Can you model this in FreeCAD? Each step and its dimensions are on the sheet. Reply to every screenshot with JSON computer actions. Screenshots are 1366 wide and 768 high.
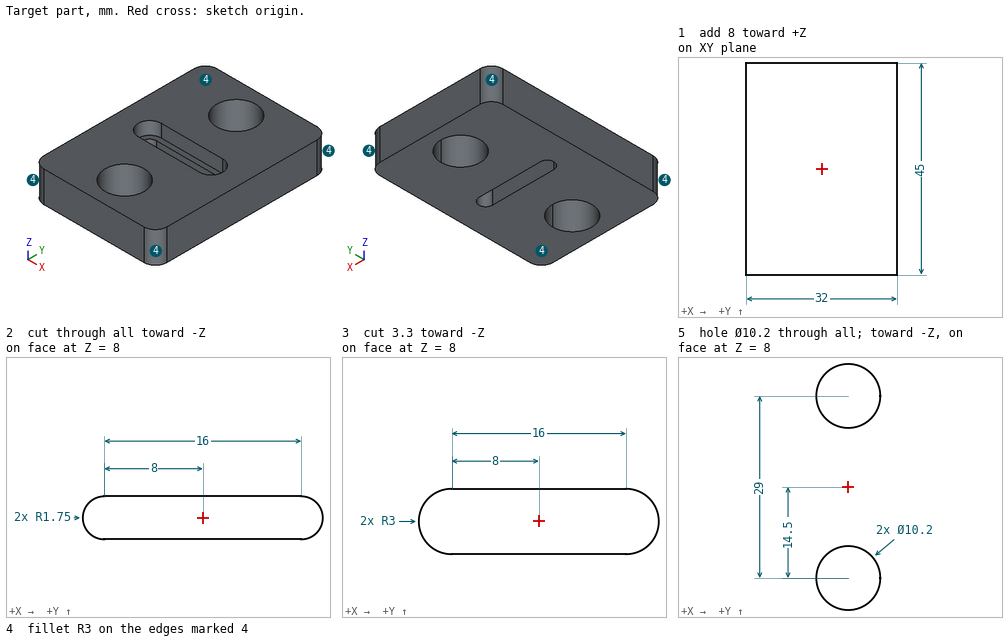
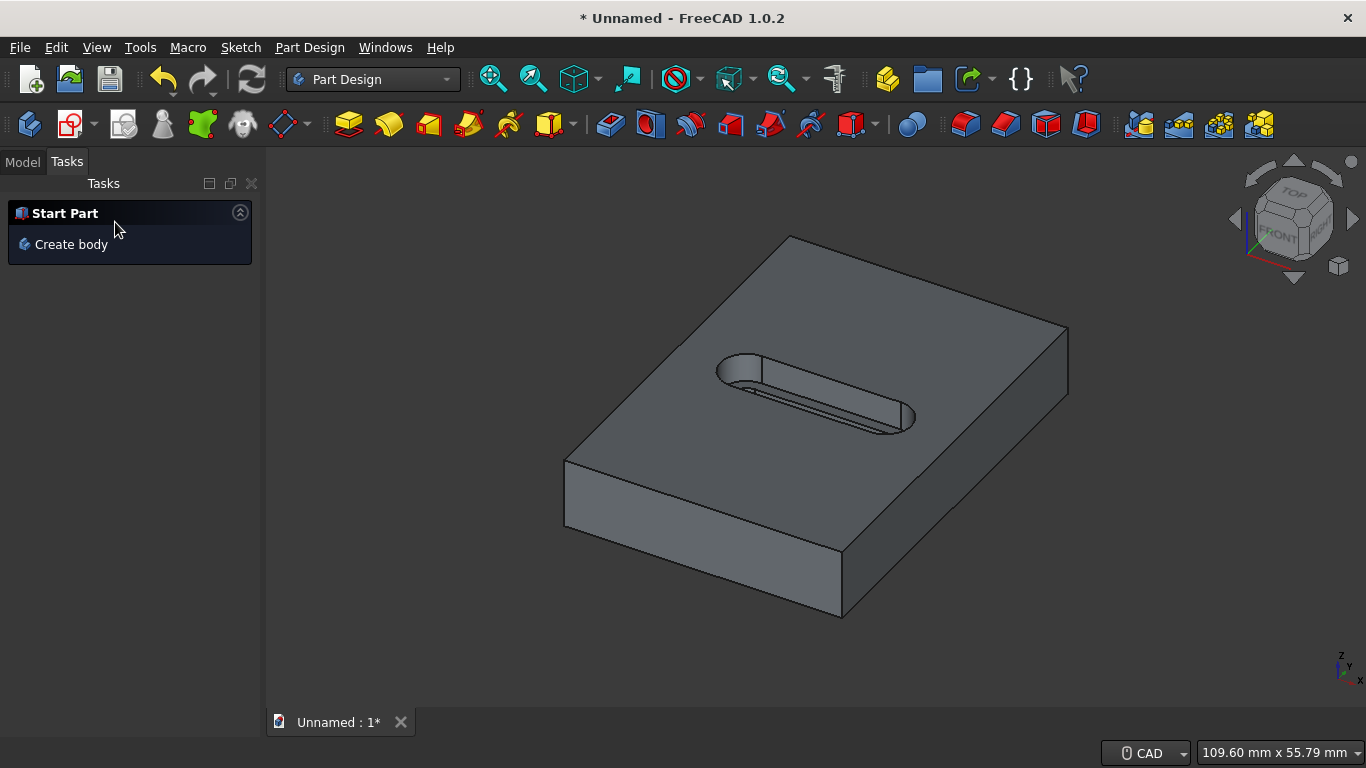
{"action": "left_click", "coordinate": [842, 584]}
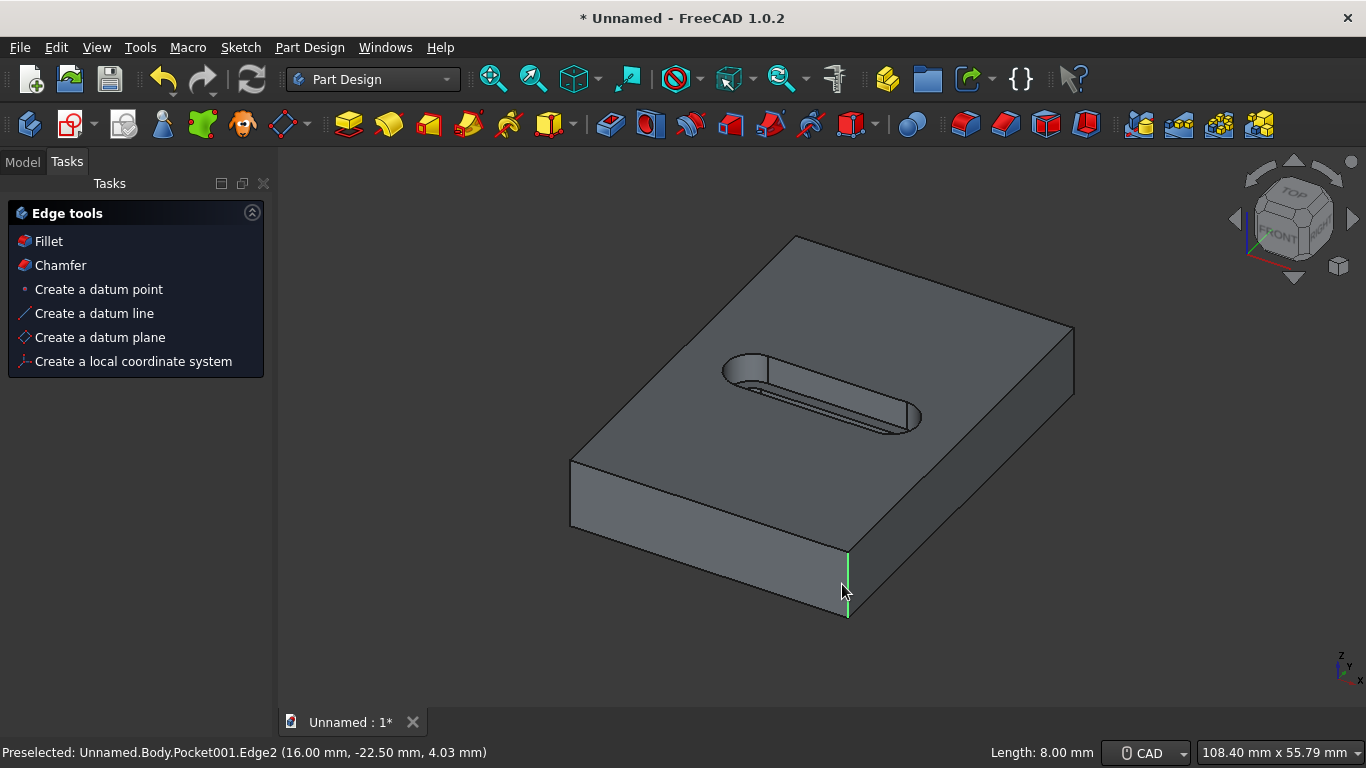
{"action": "key", "text": "0"}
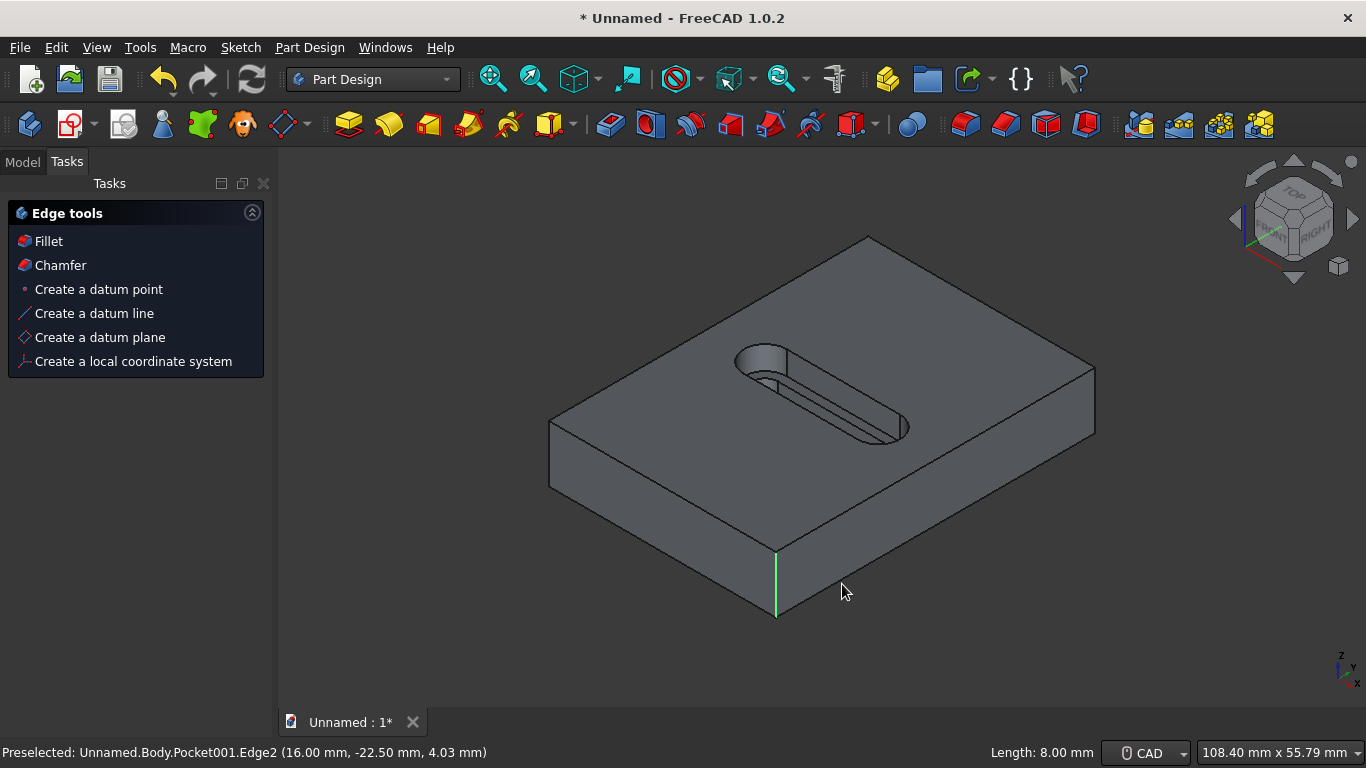
{"action": "key", "text": "2"}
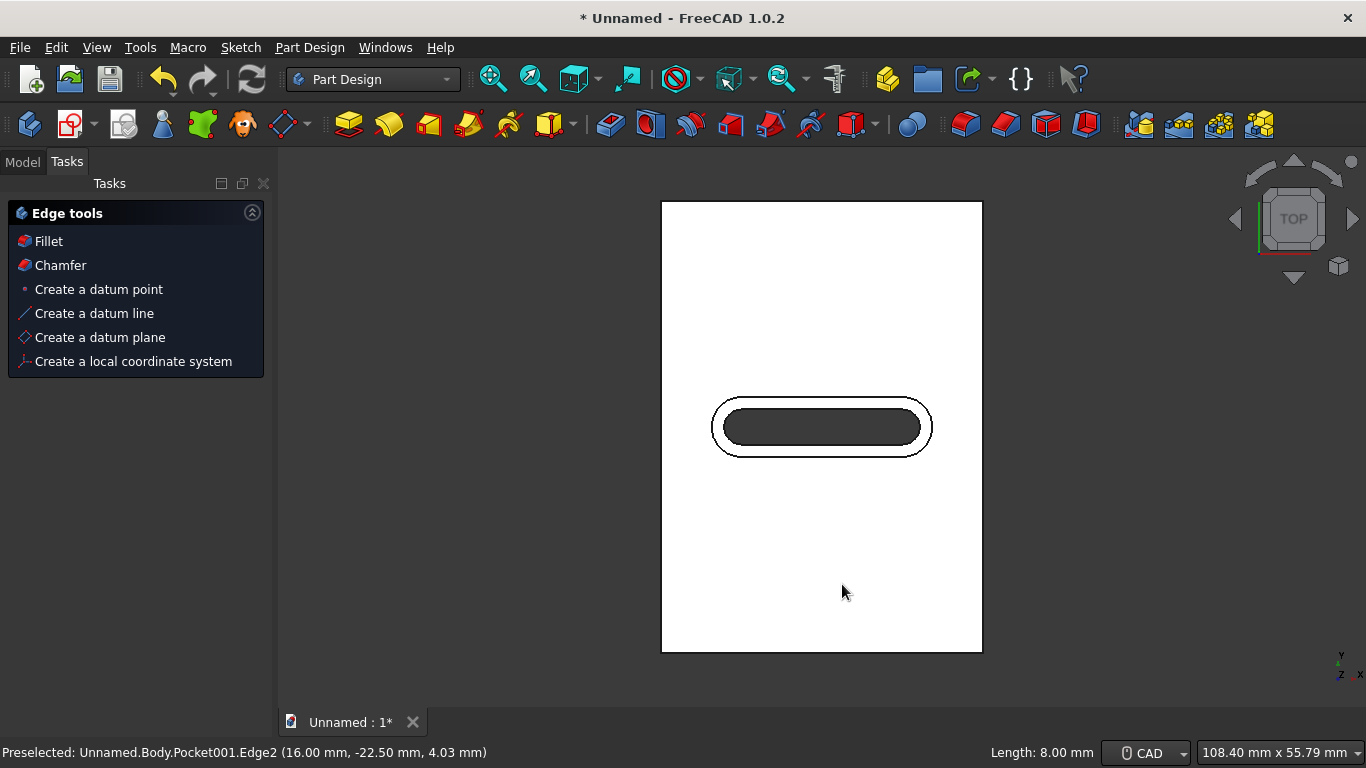
{"action": "key", "text": "1"}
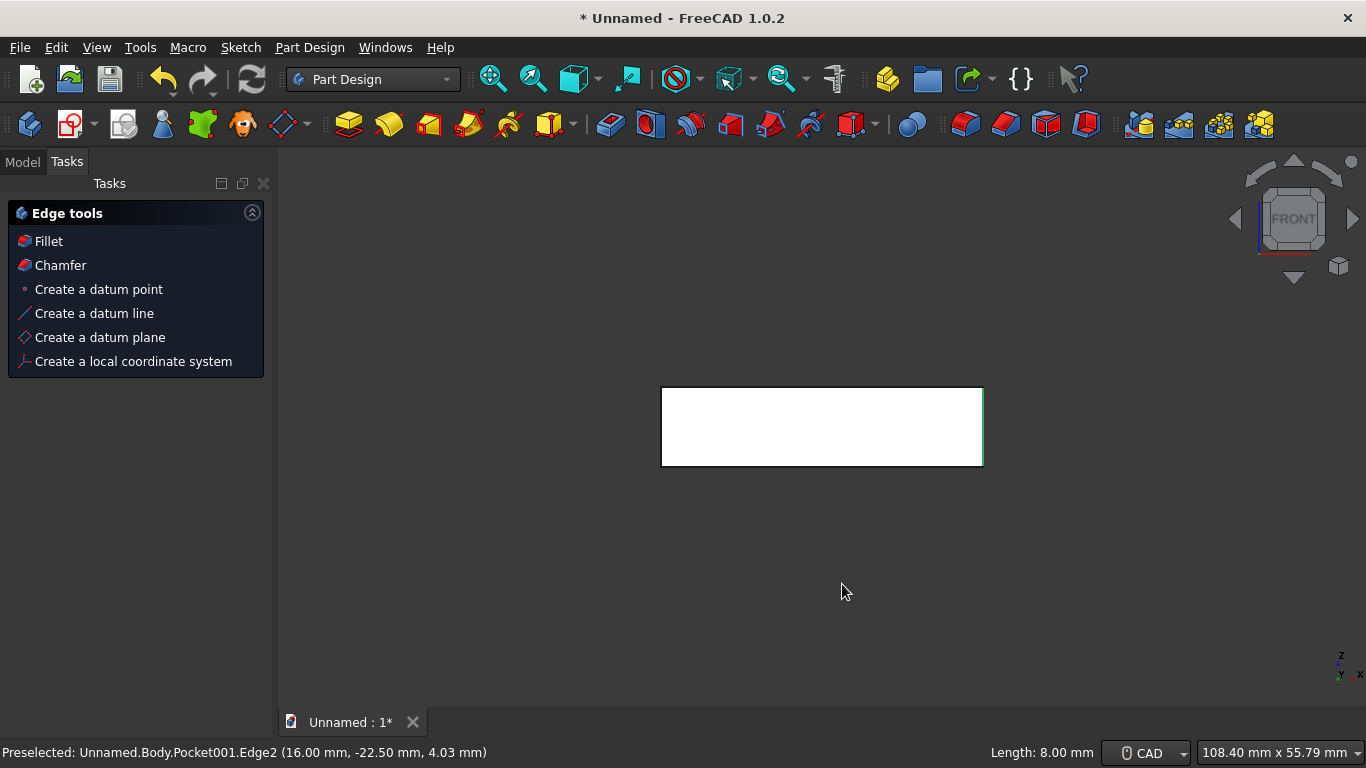
{"action": "key", "text": "v f"}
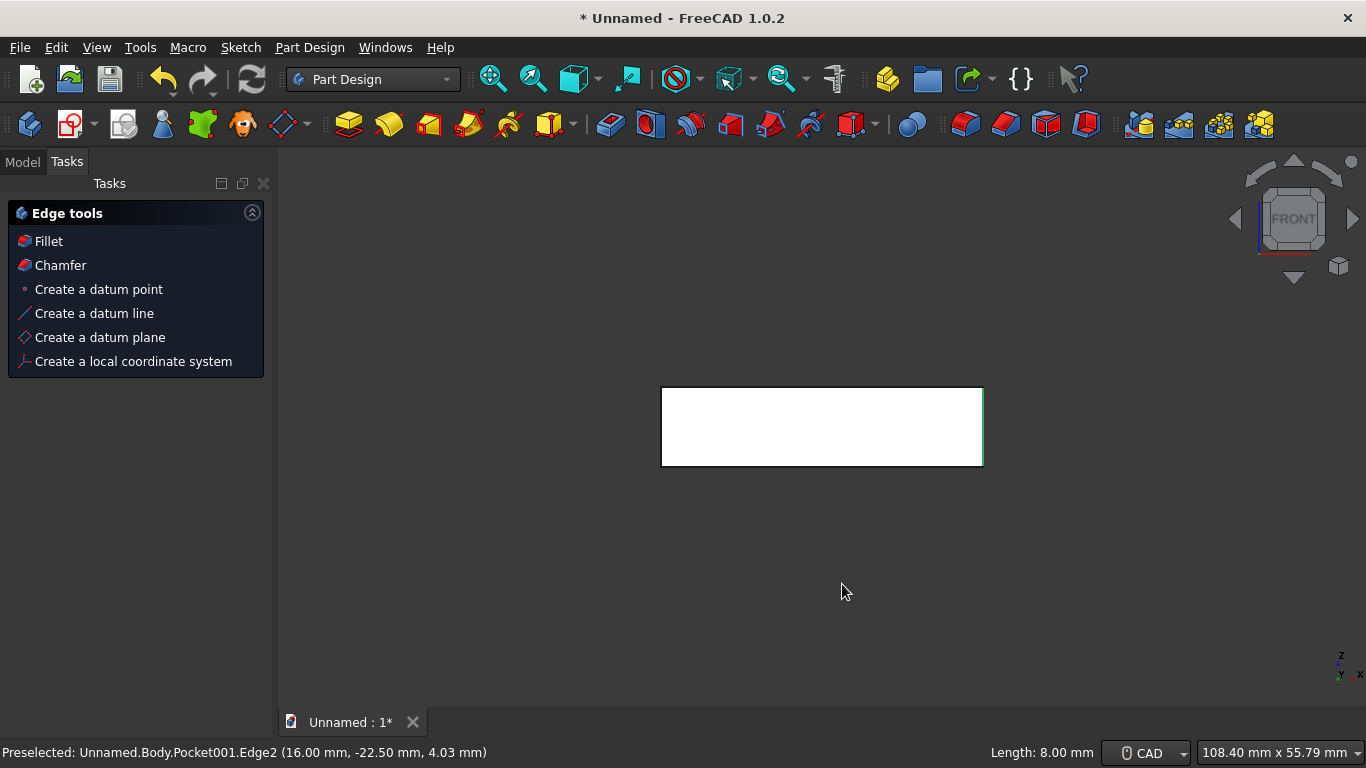
{"action": "left_click", "coordinate": [661, 426], "text": "ctrl"}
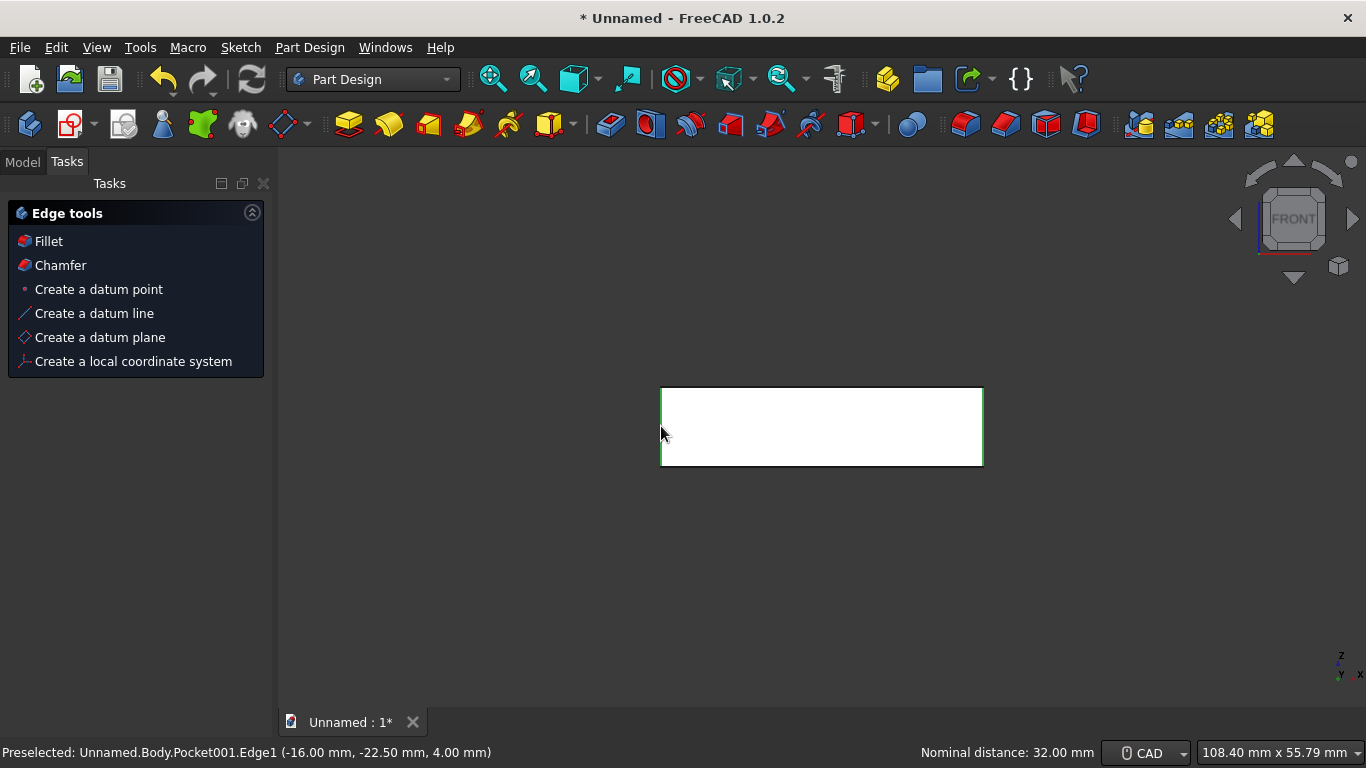
{"action": "key", "text": "3"}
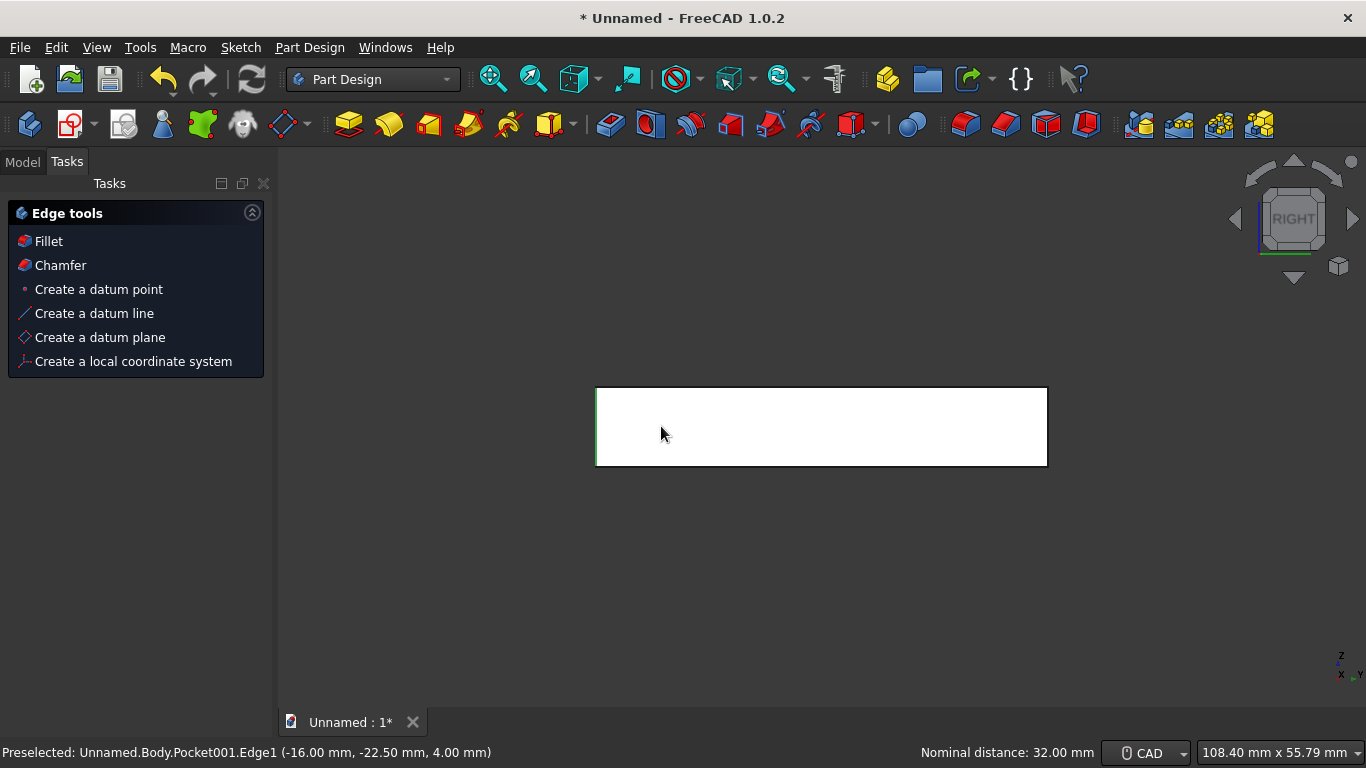
{"action": "key", "text": "v f"}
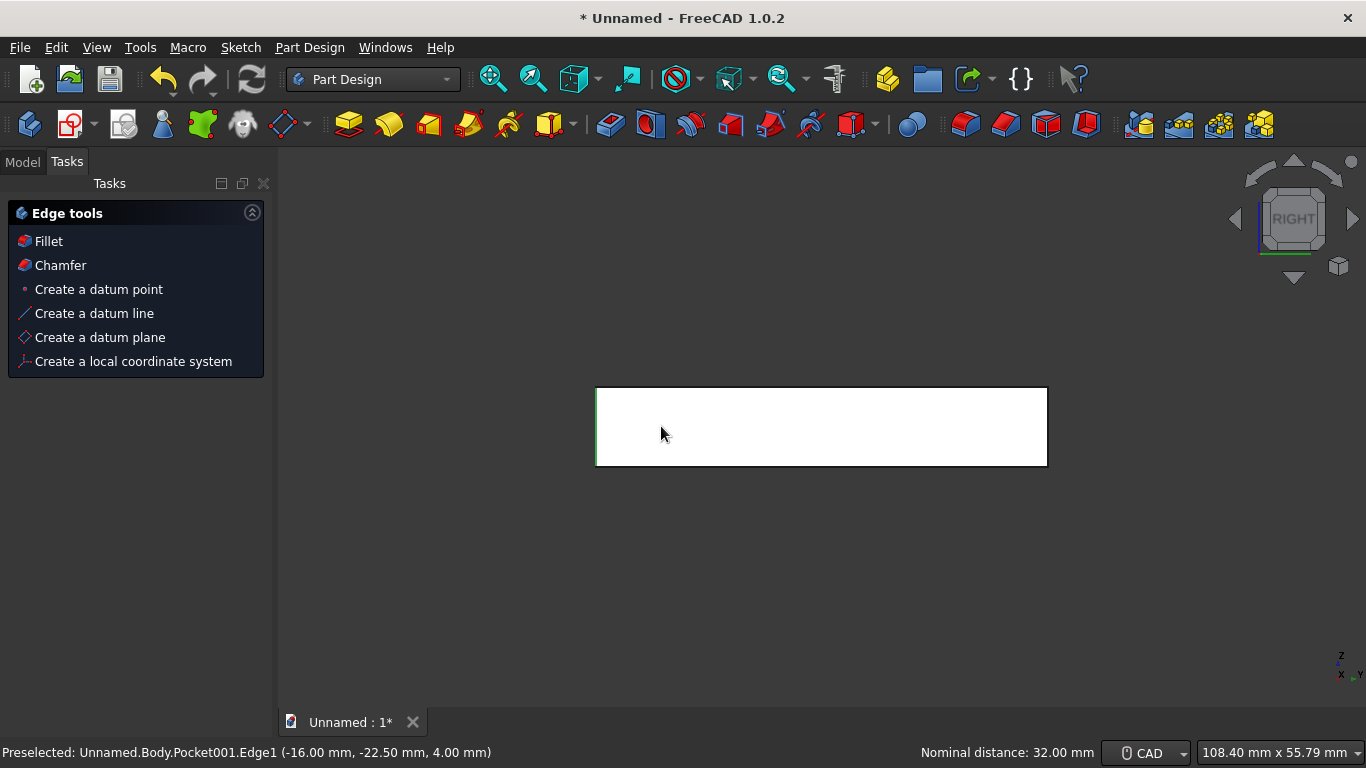
{"action": "left_click", "coordinate": [1048, 426], "text": "ctrl"}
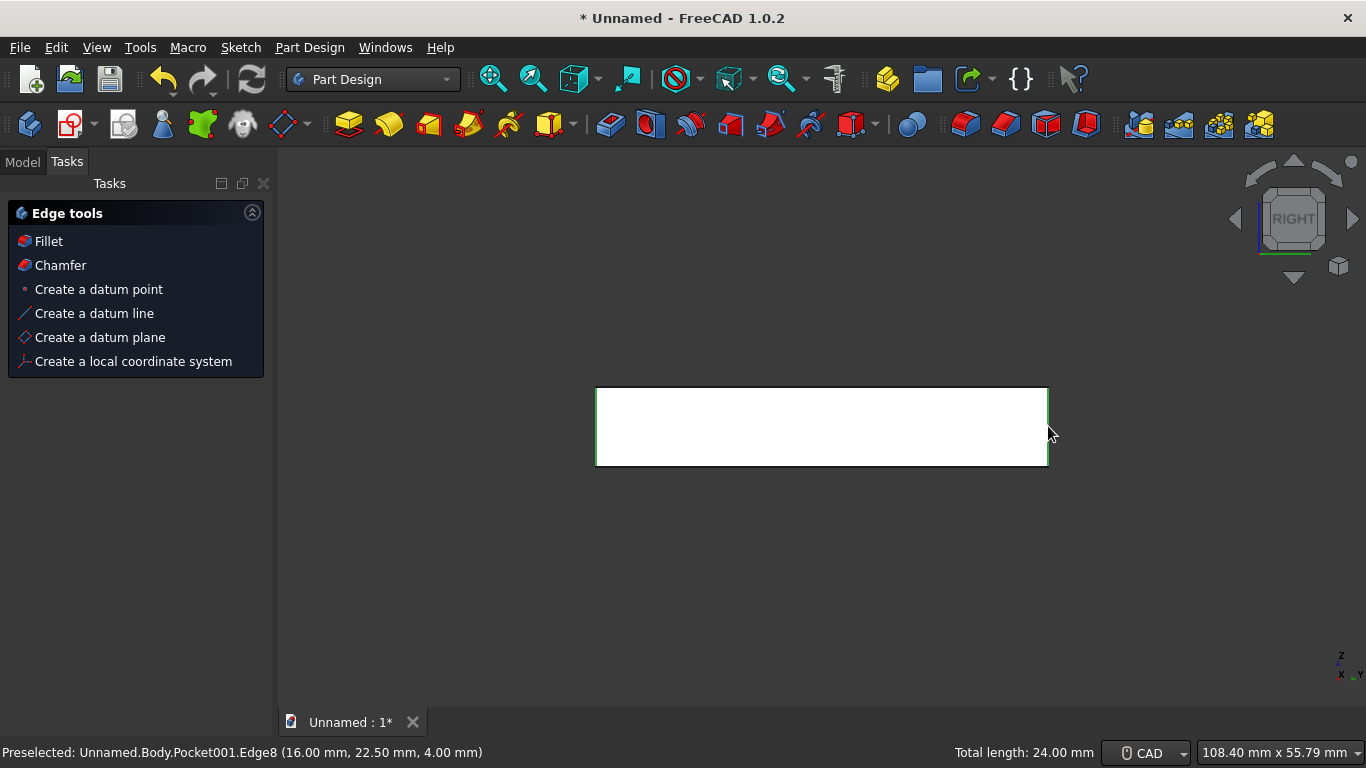
{"action": "key", "text": "5"}